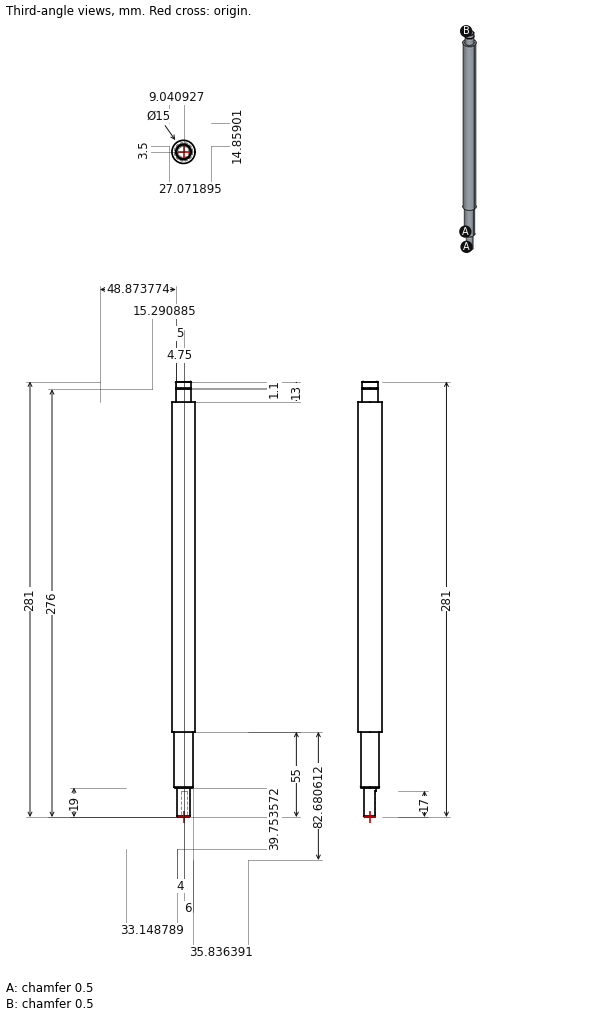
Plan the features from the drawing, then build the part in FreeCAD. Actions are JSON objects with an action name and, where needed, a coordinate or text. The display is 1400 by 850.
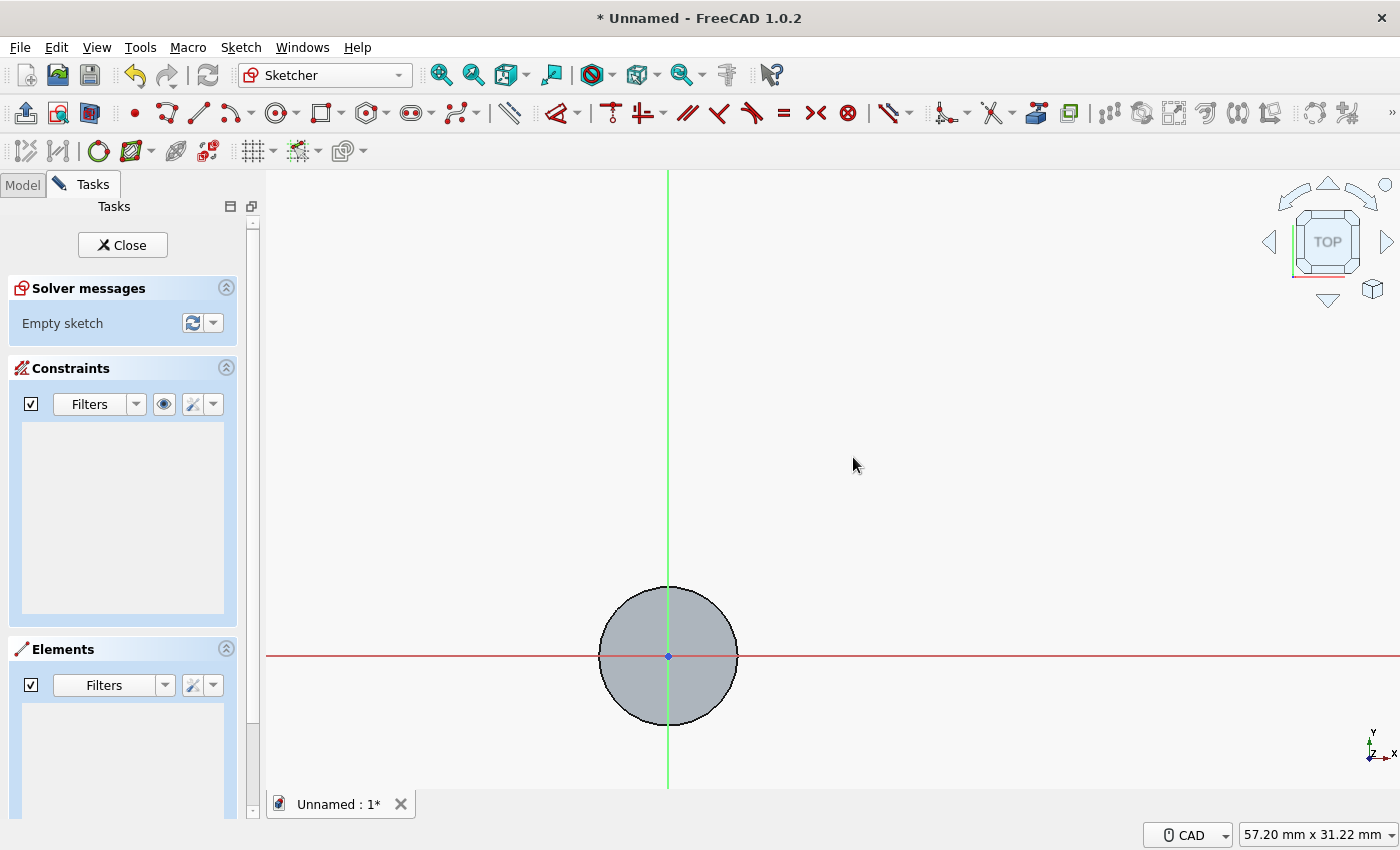
{"action": "left_click", "coordinate": [322, 114]}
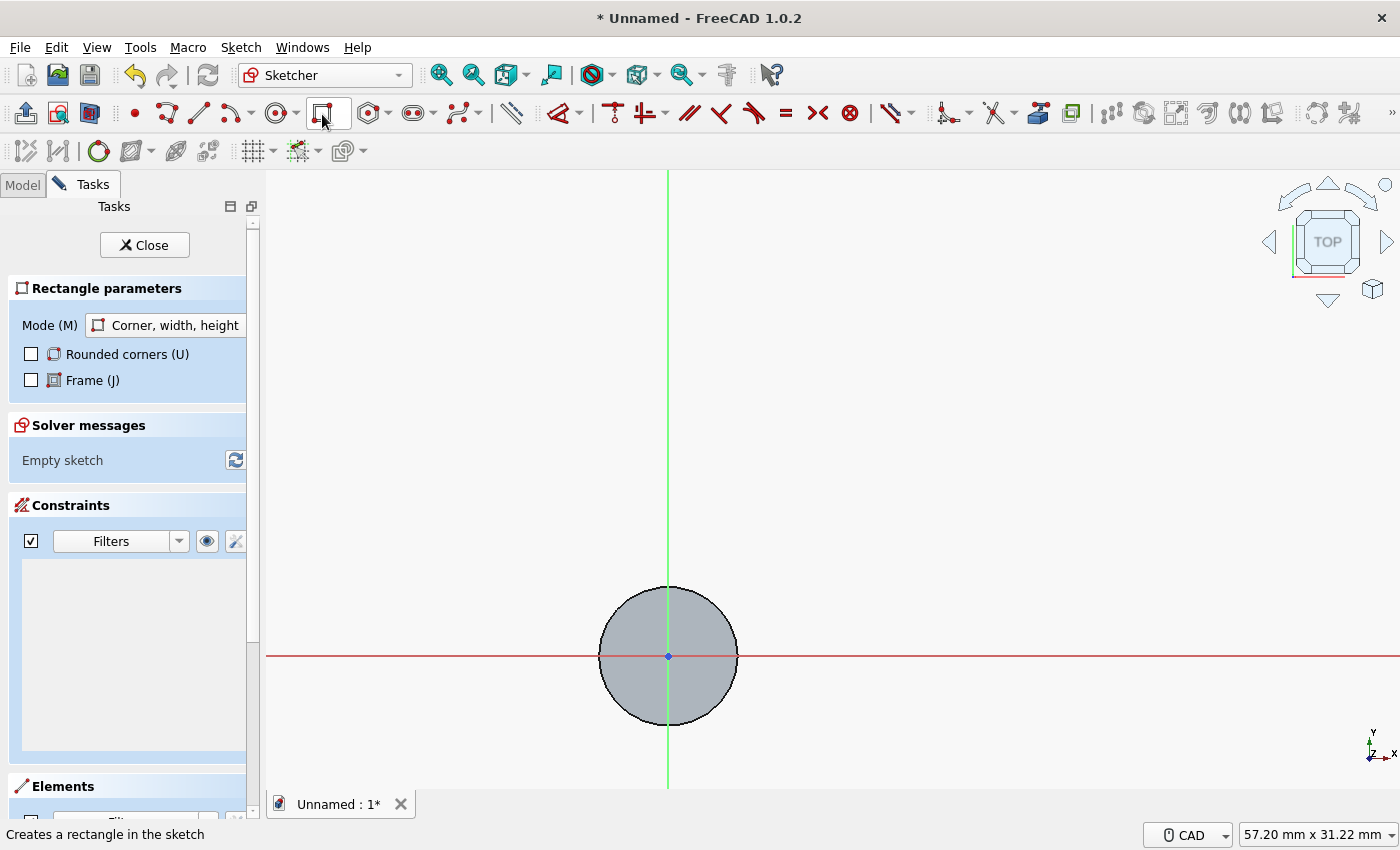
{"action": "left_click", "coordinate": [489, 292]}
{"action": "mouse_move", "coordinate": [1026, 587]}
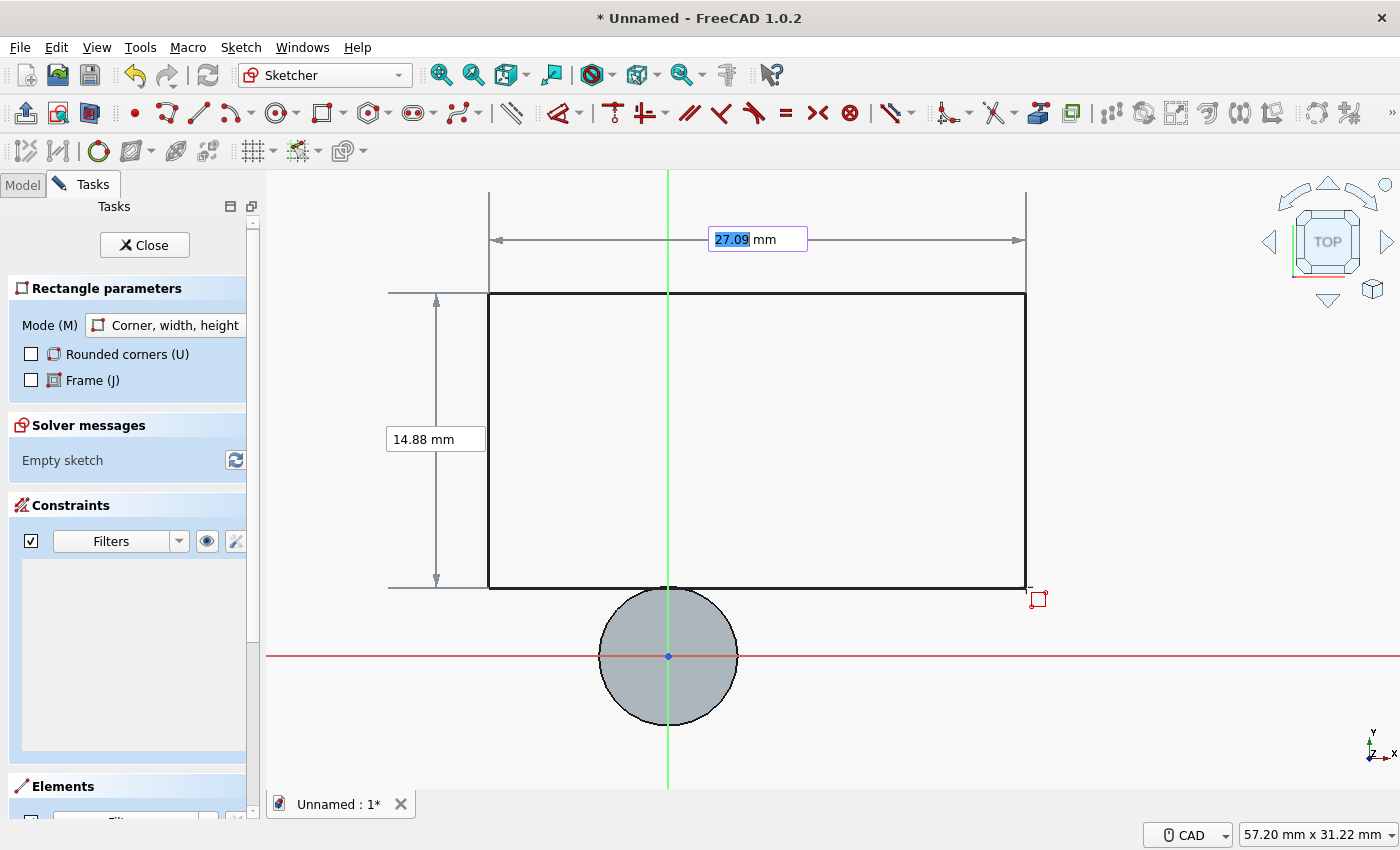
{"action": "type", "text": "27.071895"}
{"action": "key", "text": "Tab"}
{"action": "type", "text": "14.85901"}
{"action": "key", "text": "Return"}
{"action": "key", "text": "Escape"}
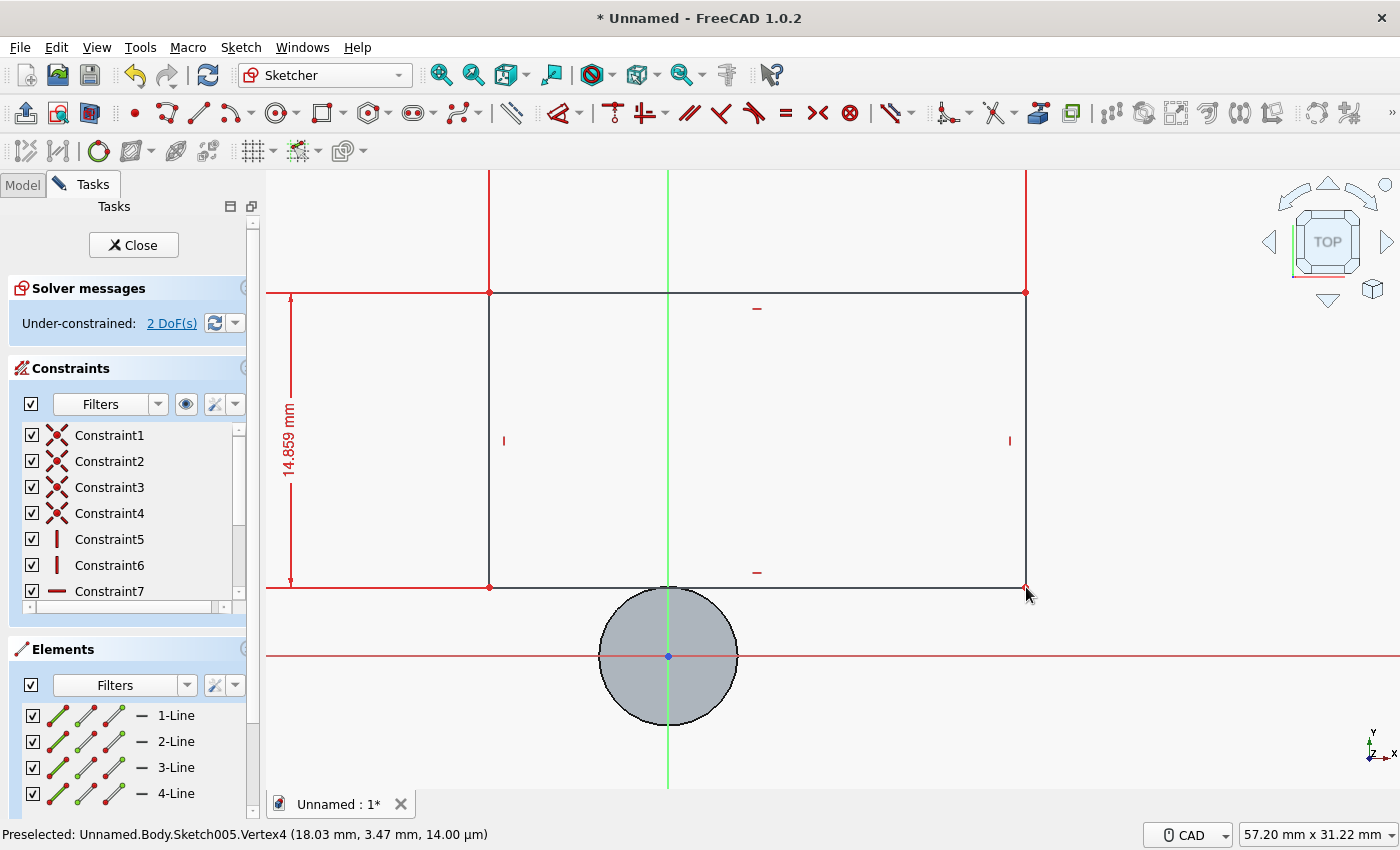
{"action": "left_click", "coordinate": [558, 114]}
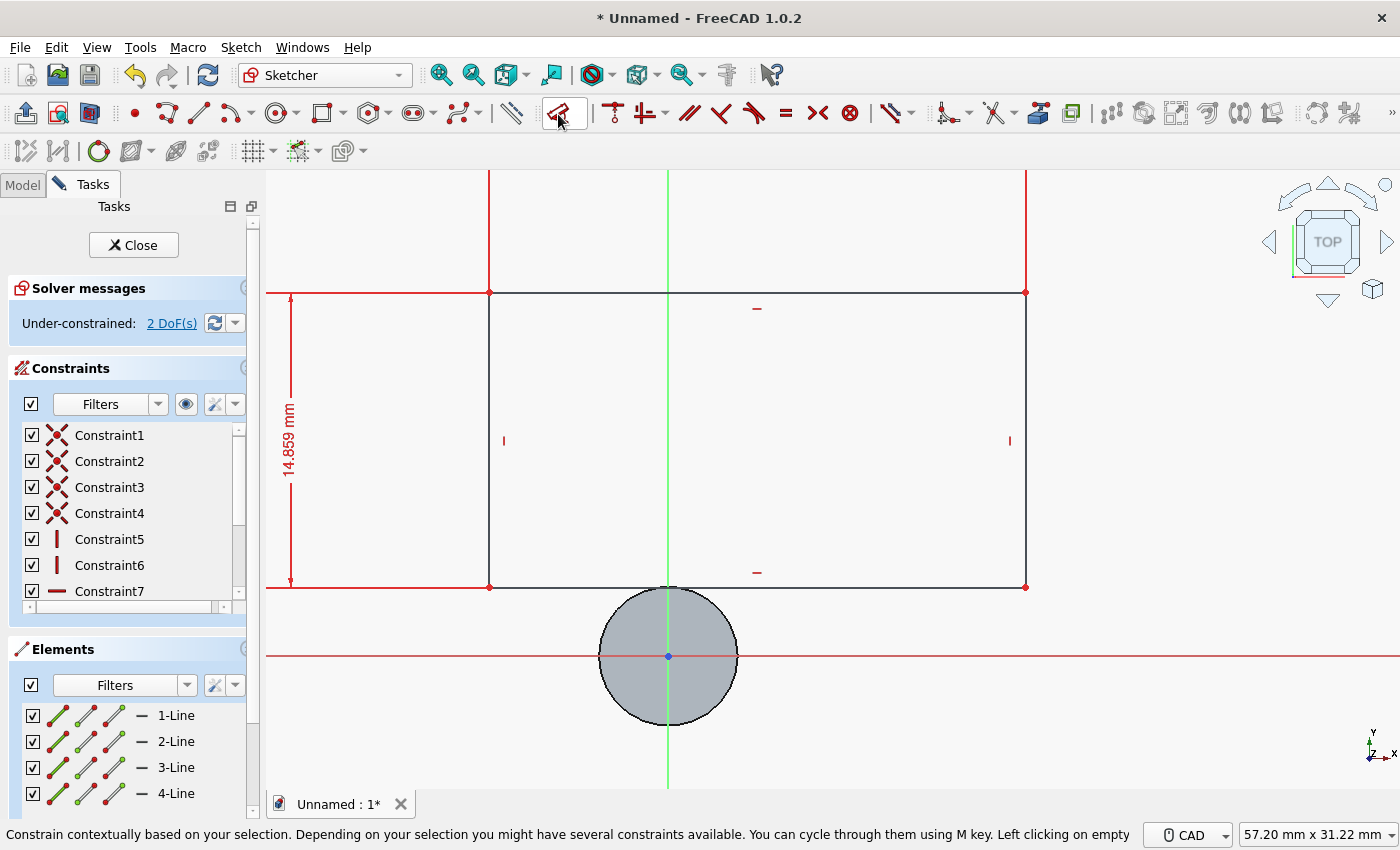
{"action": "left_click", "coordinate": [489, 588]}
{"action": "left_click", "coordinate": [455, 622]}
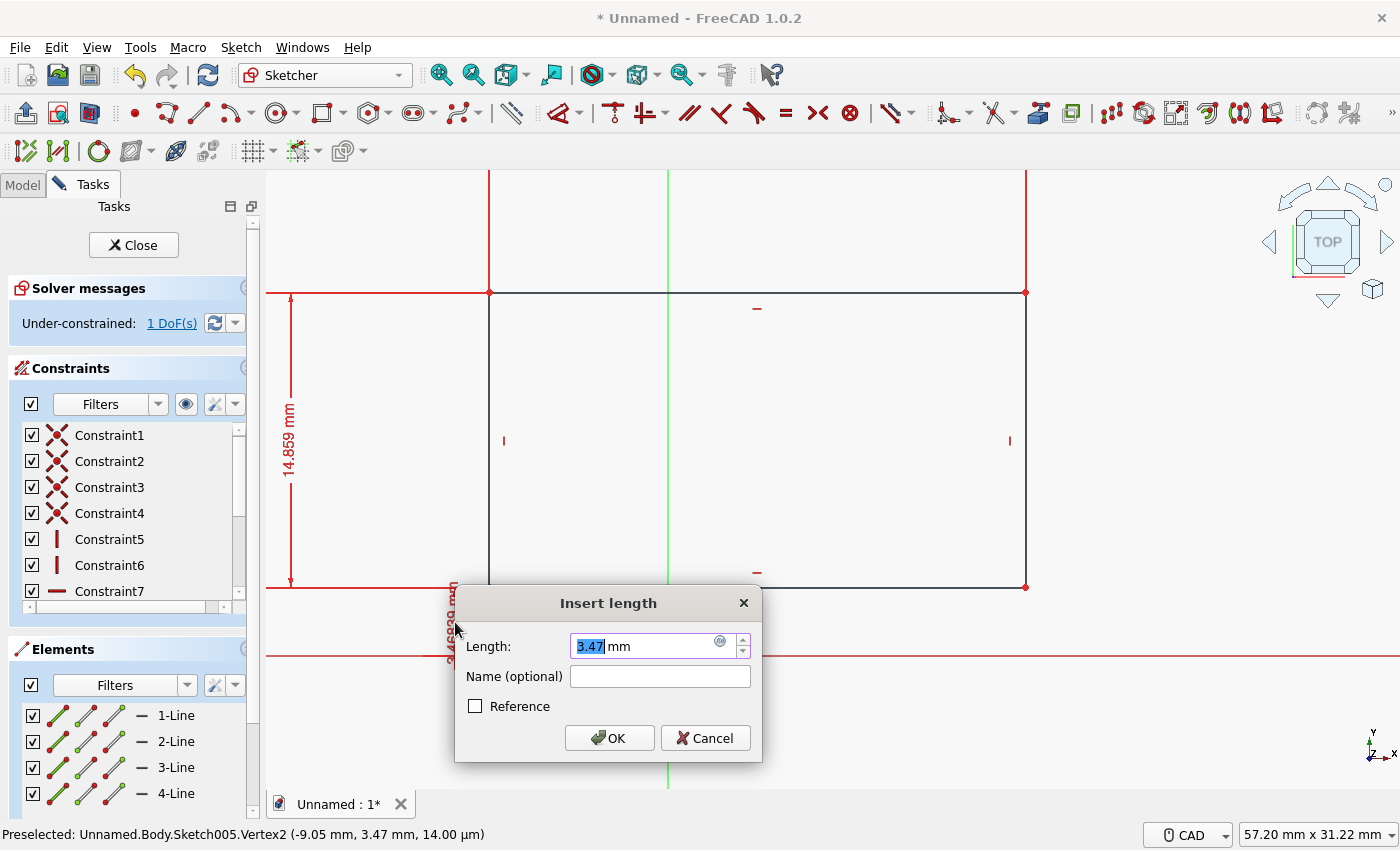
{"action": "type", "text": "3.5"}
{"action": "key", "text": "Return"}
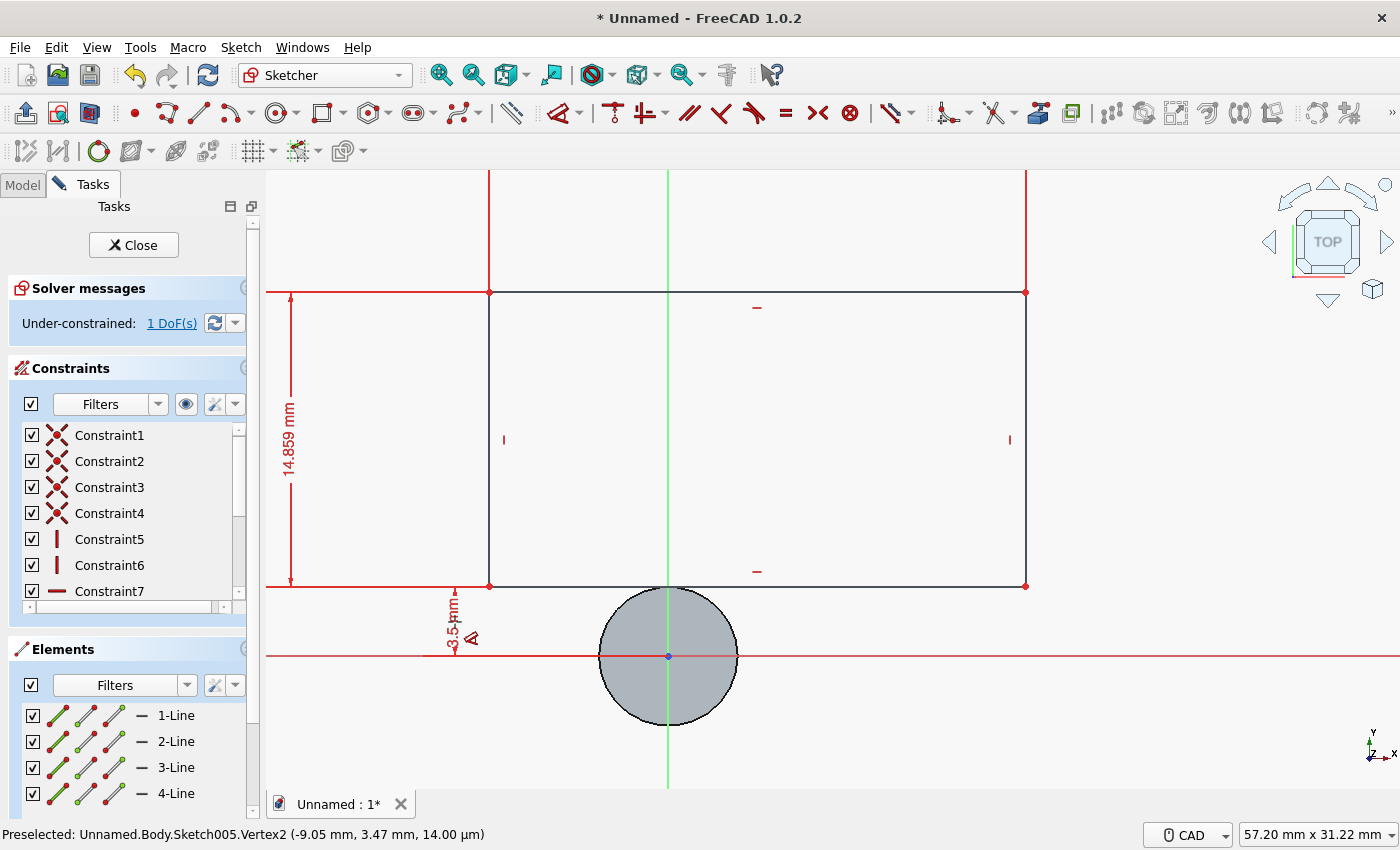
{"action": "left_click", "coordinate": [489, 292]}
{"action": "left_click", "coordinate": [579, 690]}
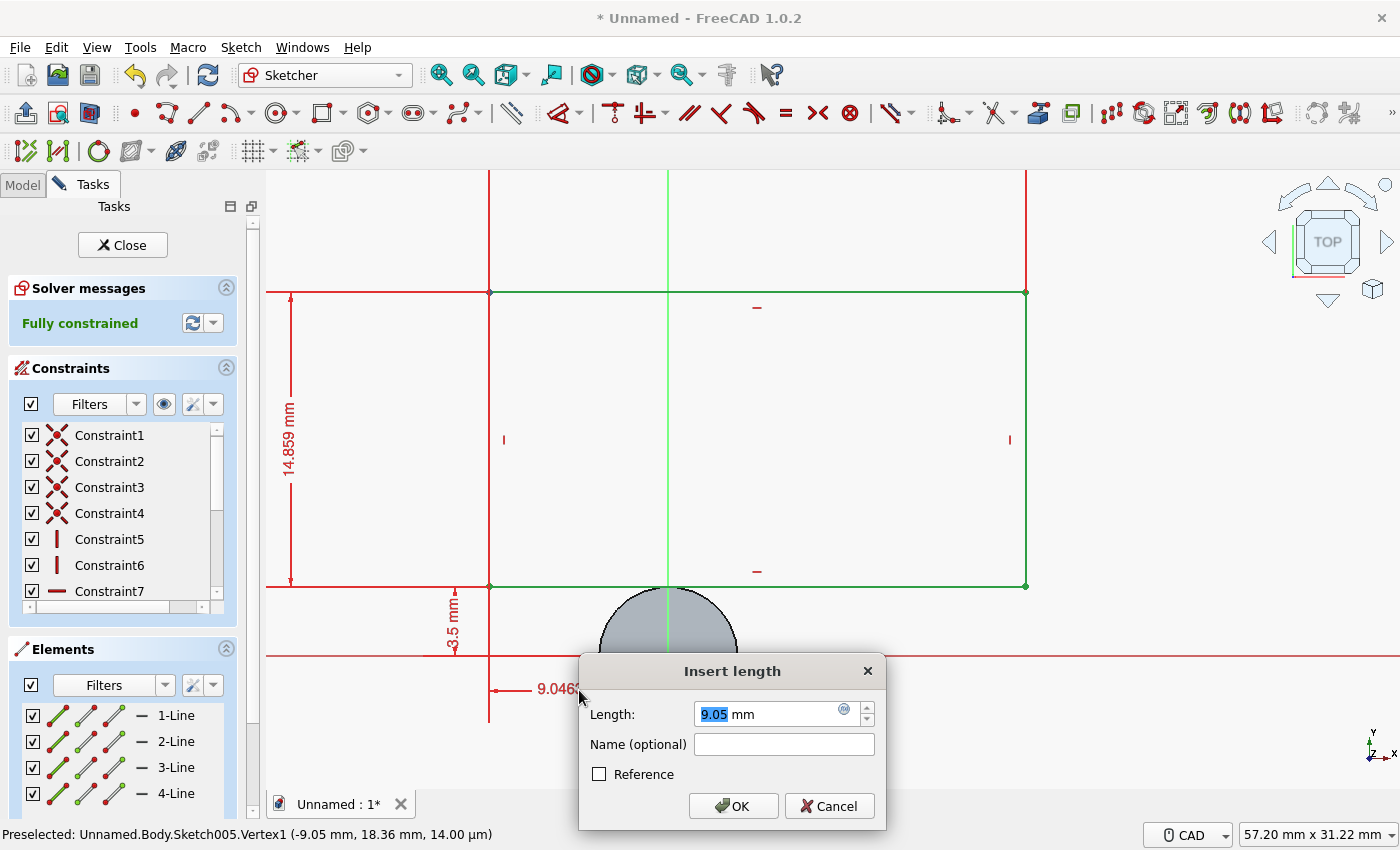
{"action": "type", "text": "9.040927"}
{"action": "key", "text": "Return"}
{"action": "key", "text": "Escape"}